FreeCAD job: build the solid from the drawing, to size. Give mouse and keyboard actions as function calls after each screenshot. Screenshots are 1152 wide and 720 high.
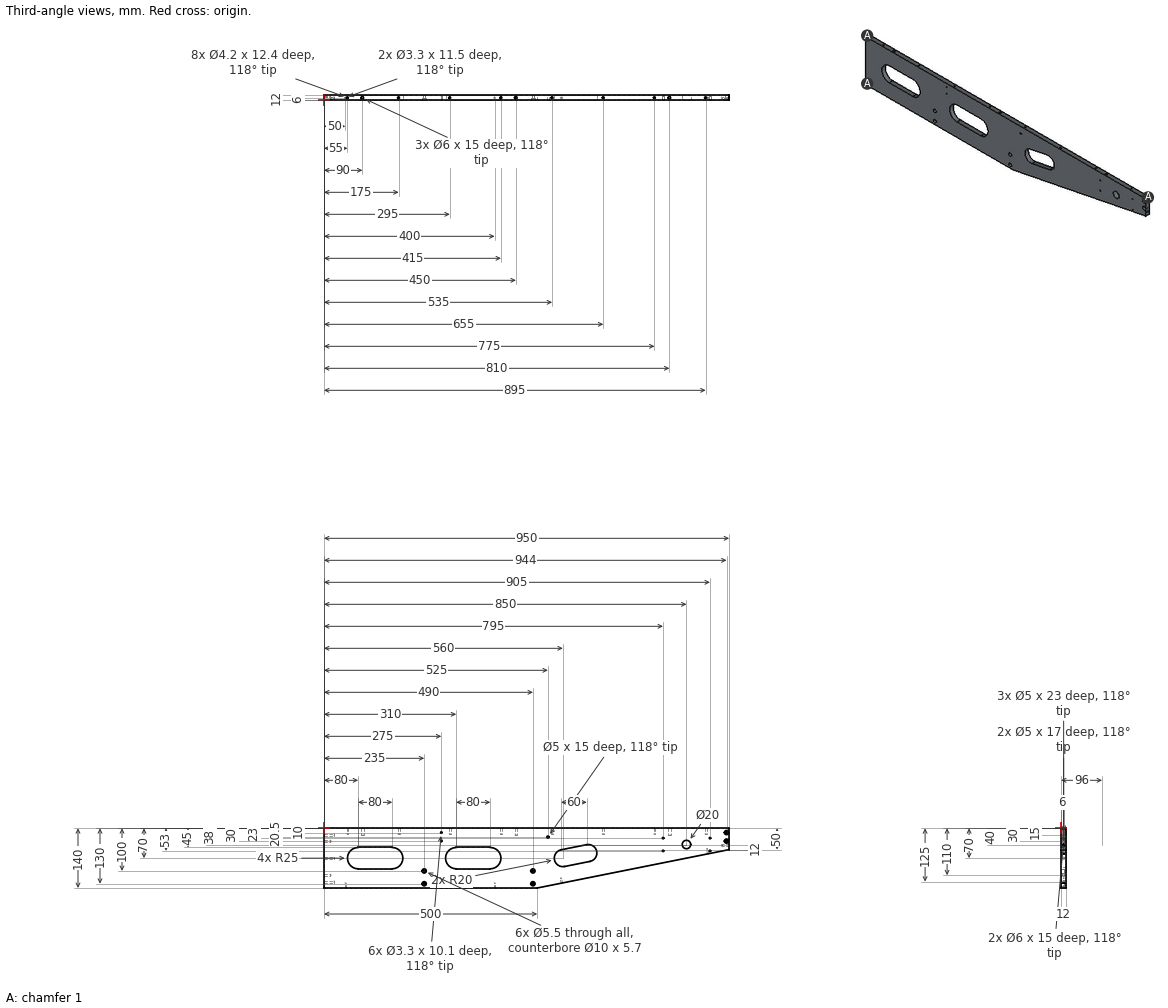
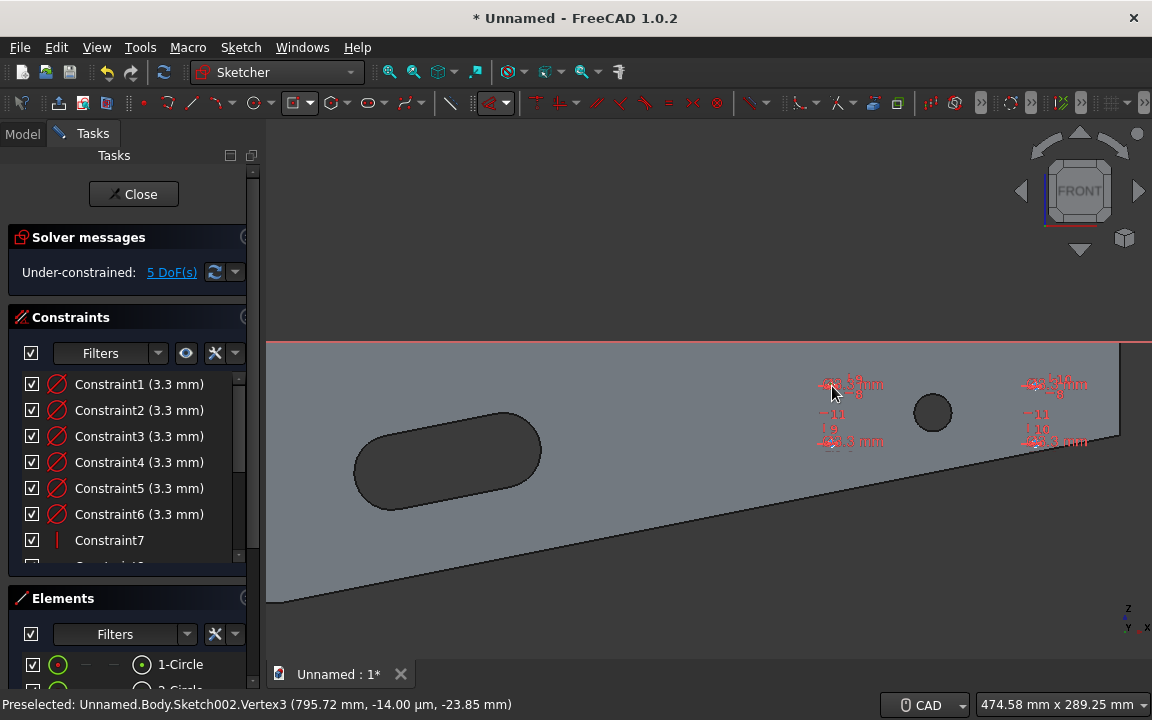
key(i)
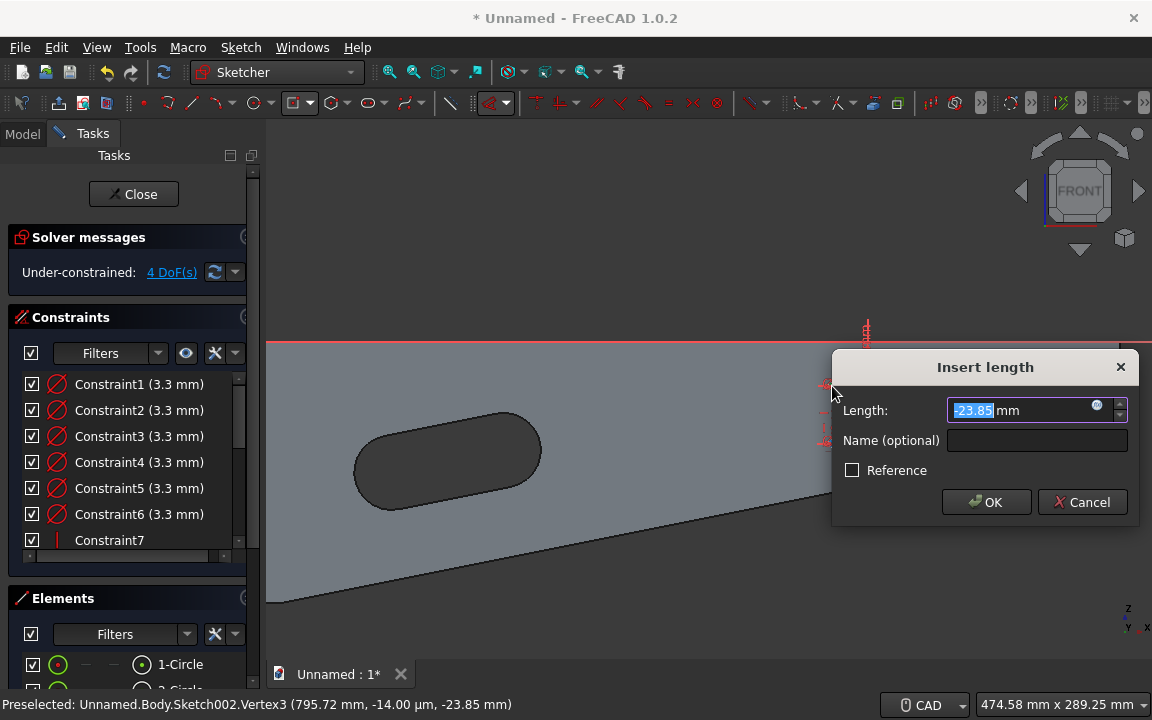
text(-23)
key(Return)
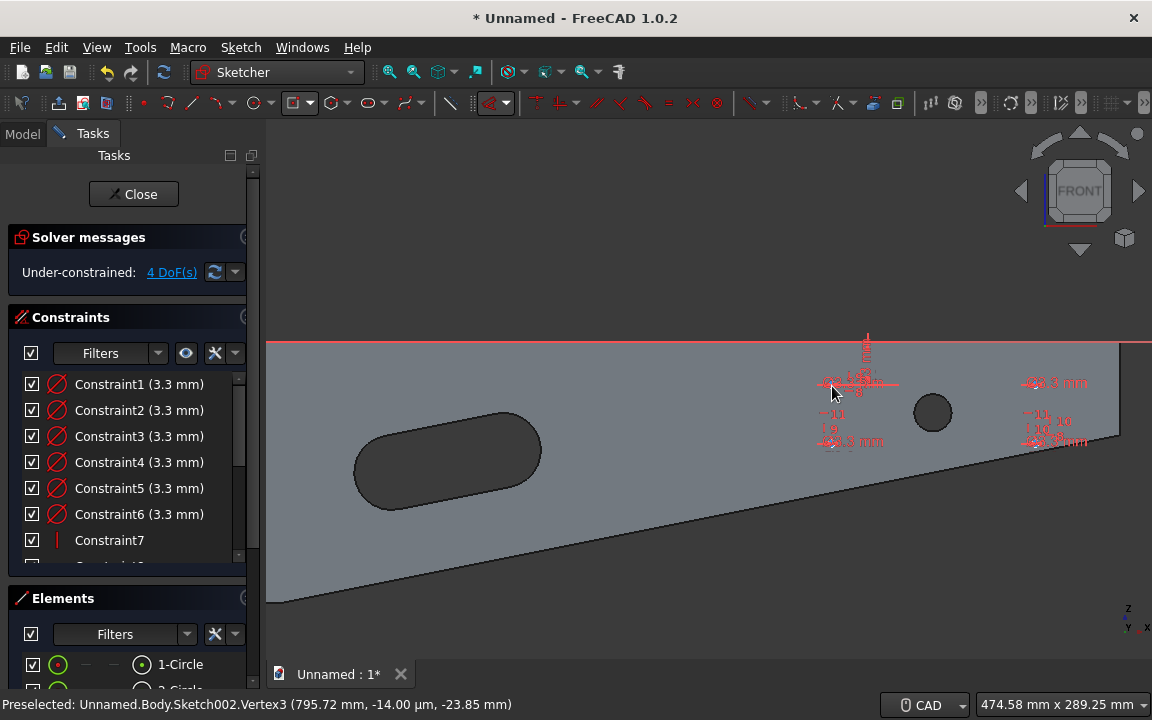
click(832, 444)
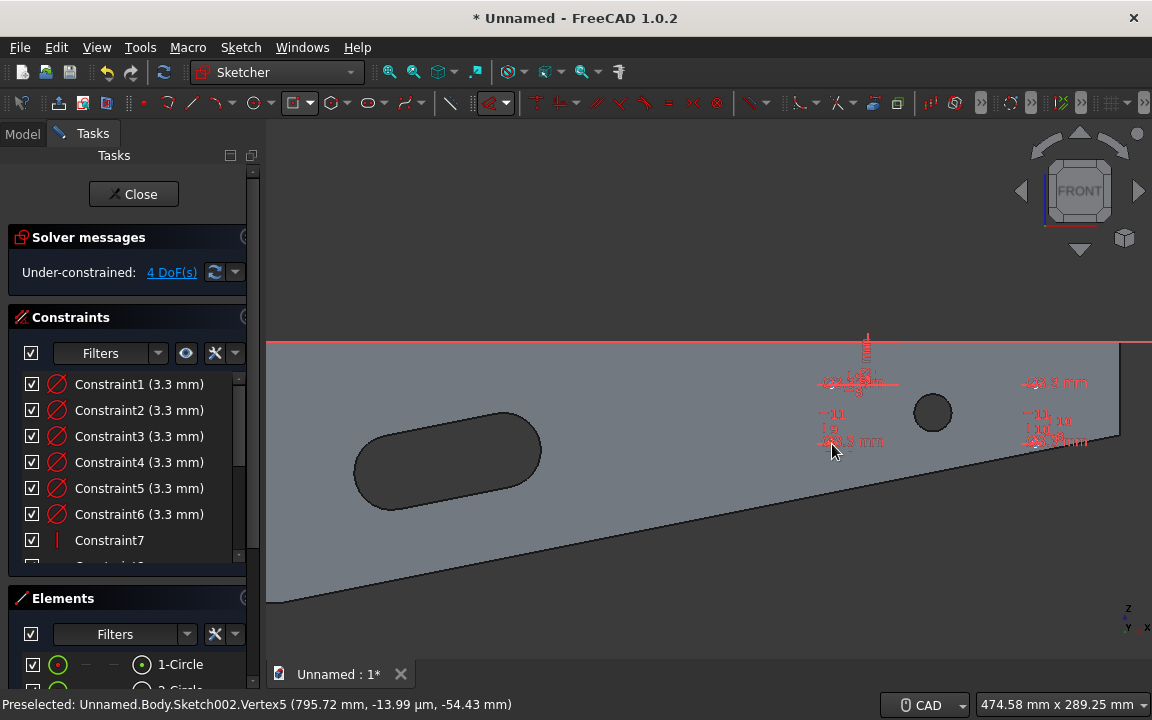
key(i)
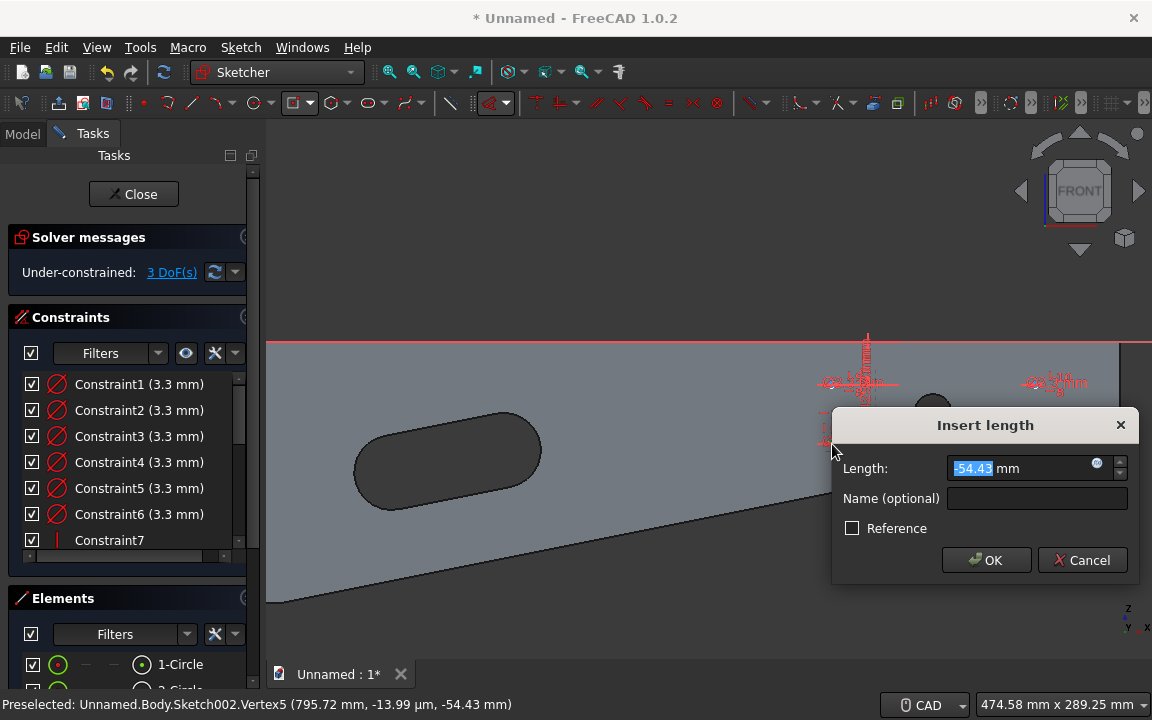
text(-53)
key(Return)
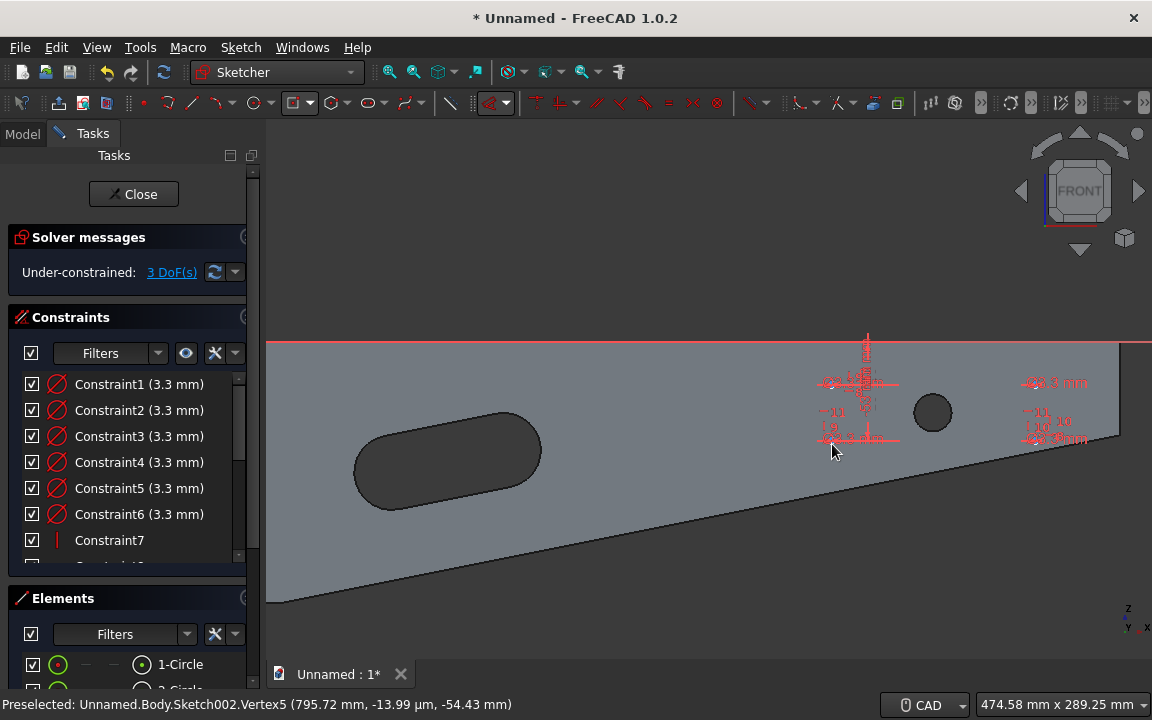
scroll(834, 387, down, 6)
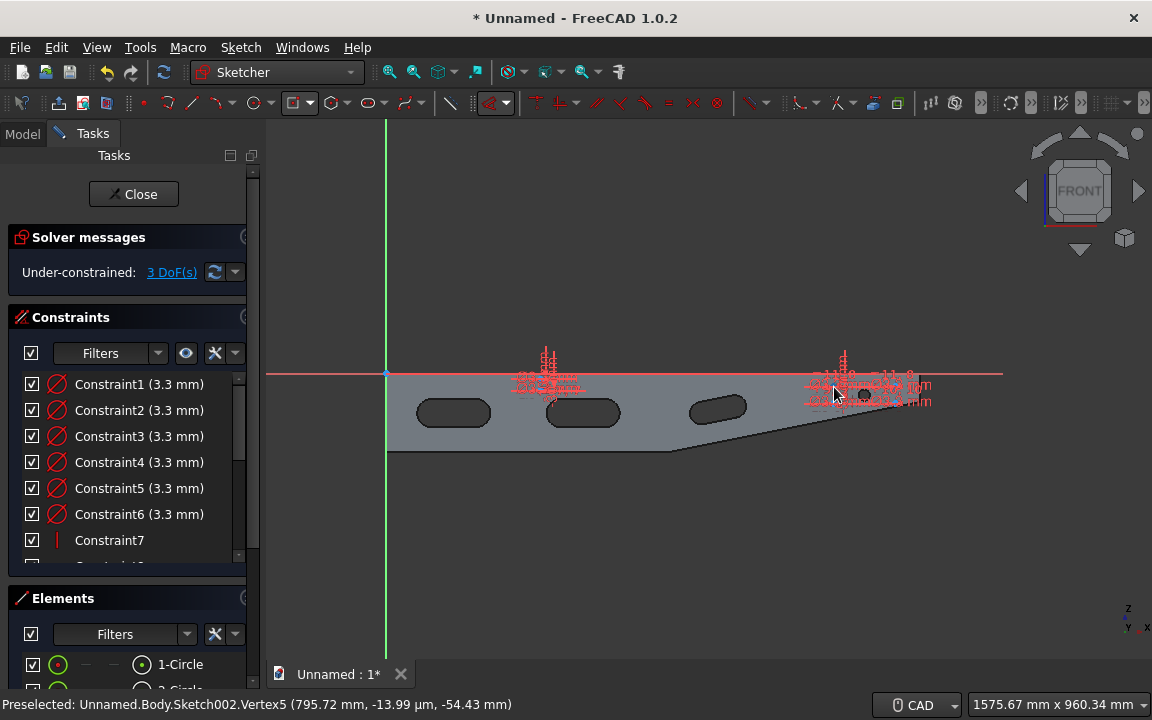
click(541, 379)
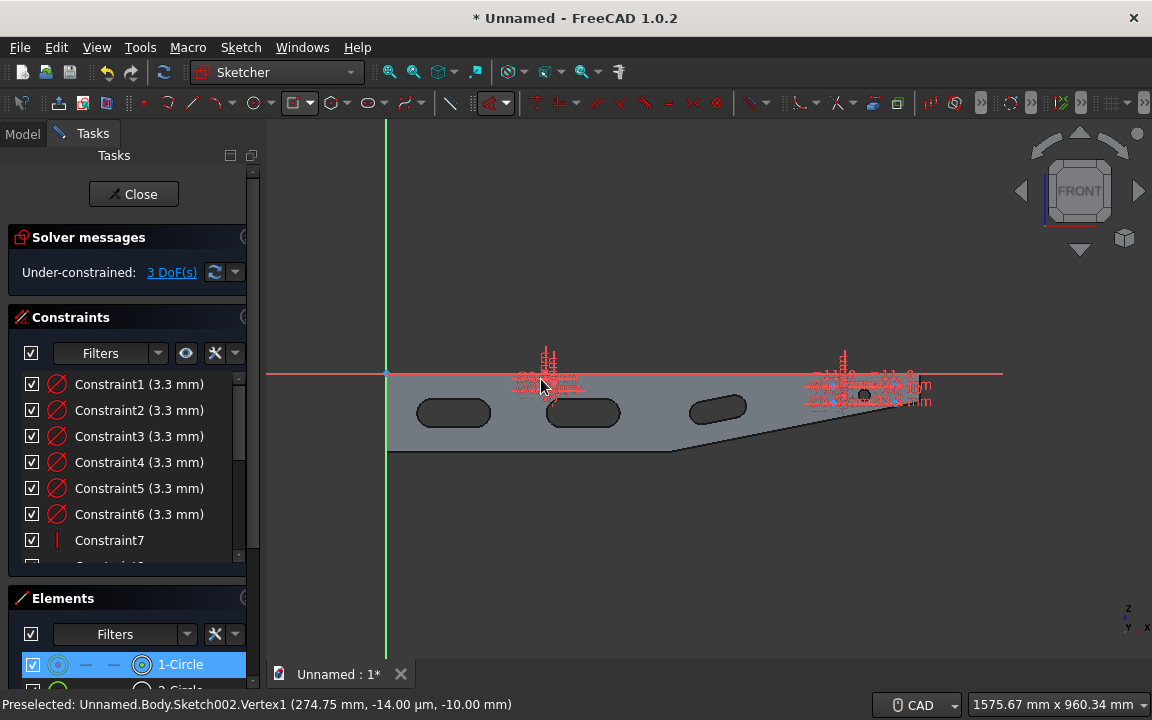
key(l)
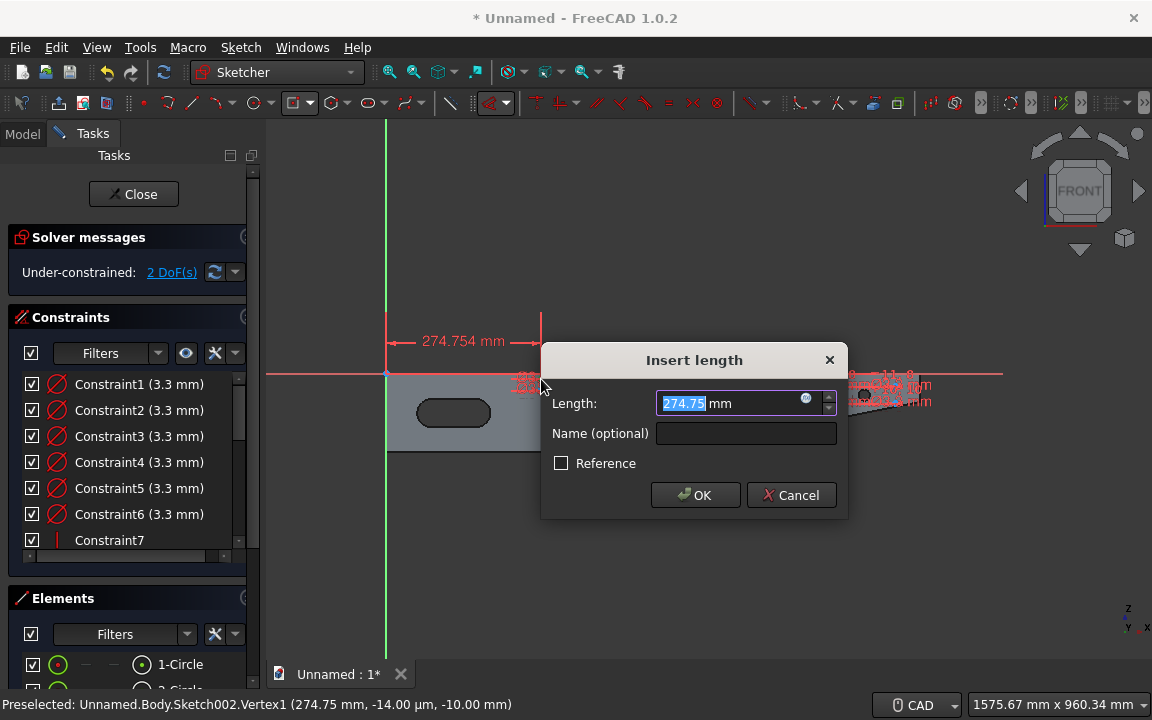
text(275)
key(Return)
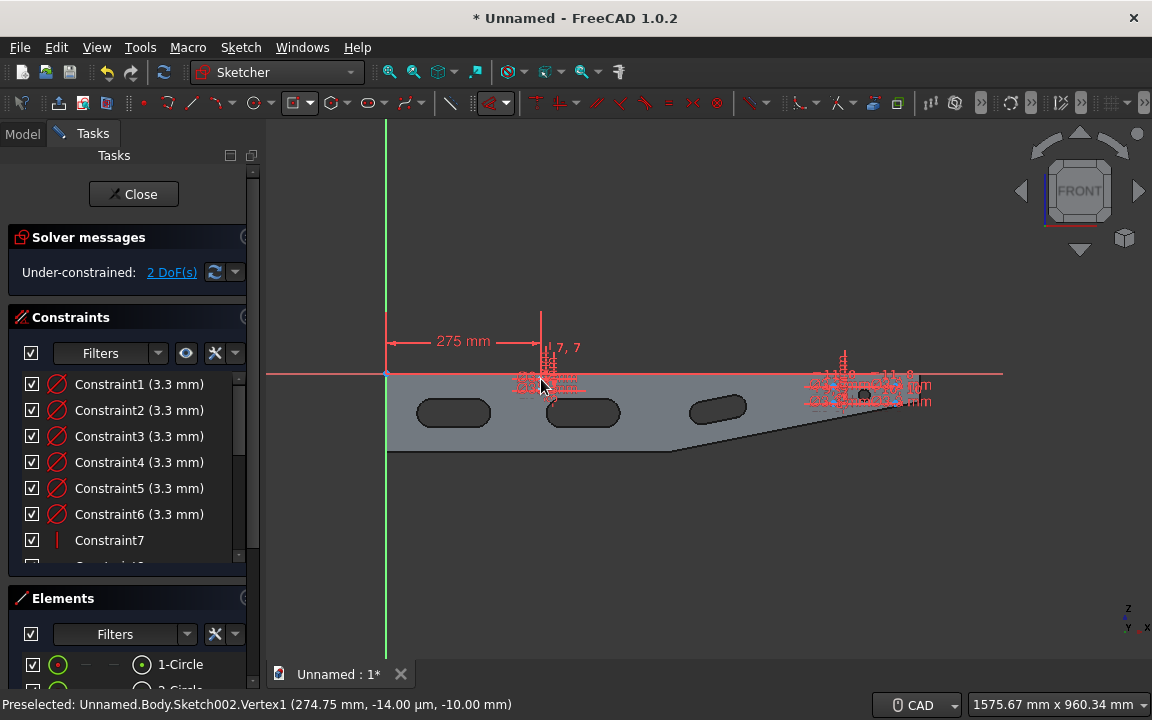
click(834, 387)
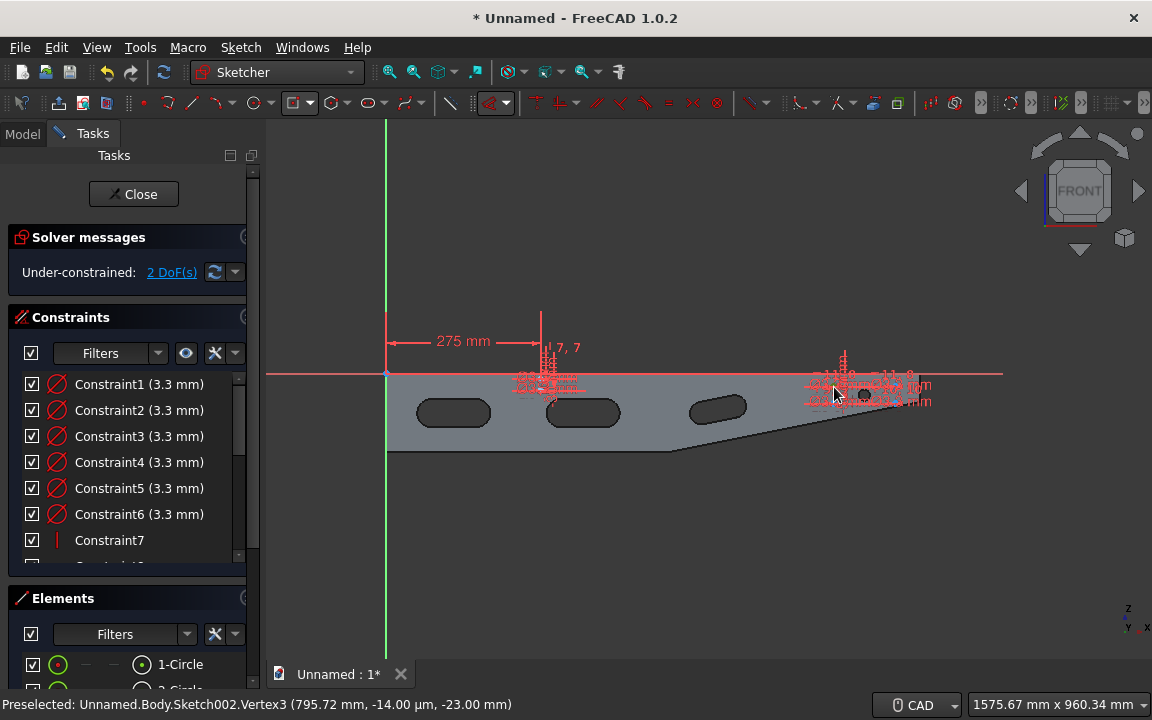
key(l)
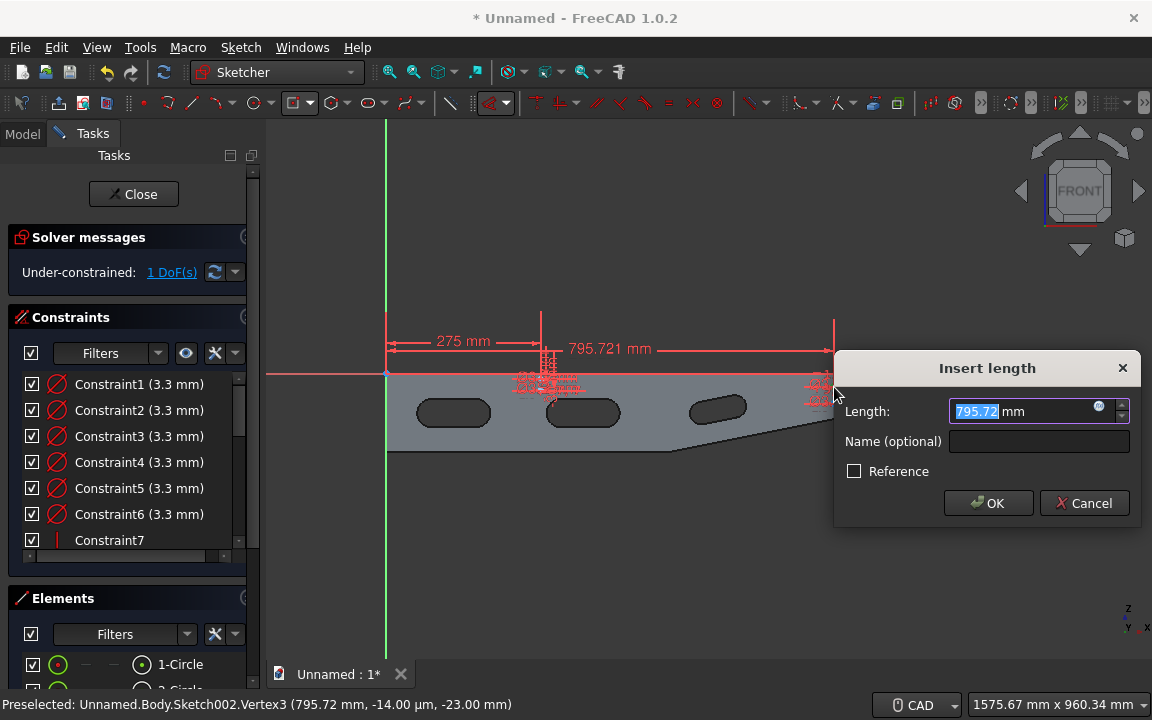
text(795)
key(Return)